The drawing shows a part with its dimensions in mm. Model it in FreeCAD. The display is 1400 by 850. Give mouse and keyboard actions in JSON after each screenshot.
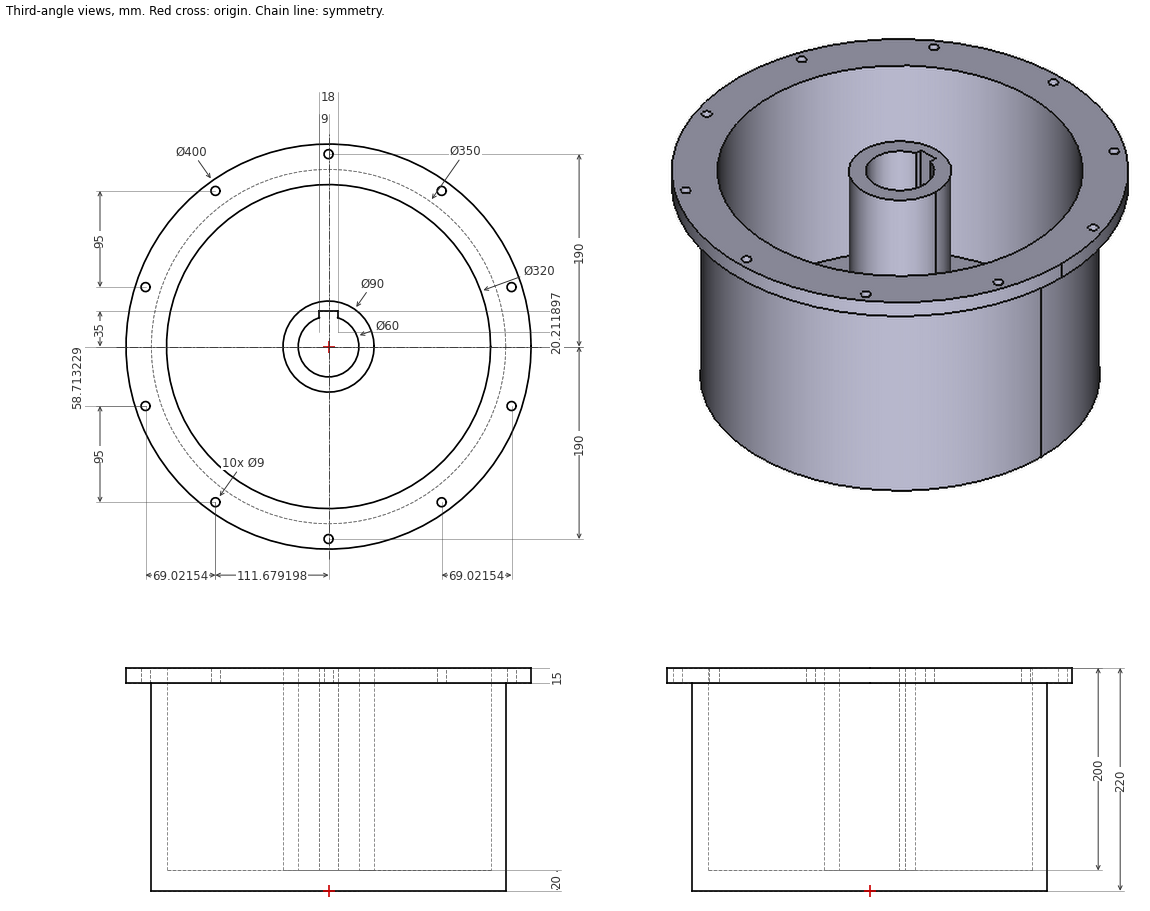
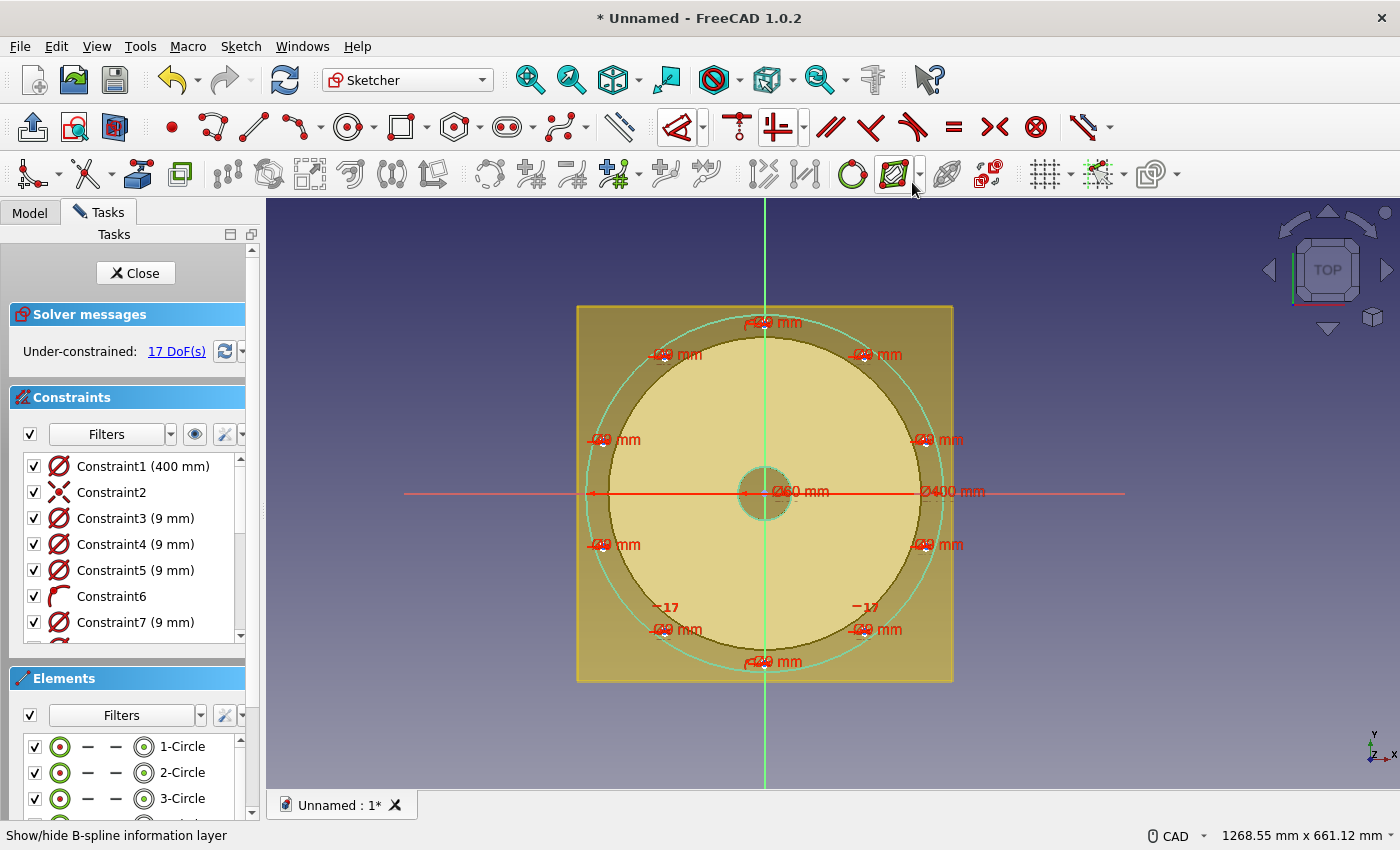
{"action": "left_click", "coordinate": [603, 547]}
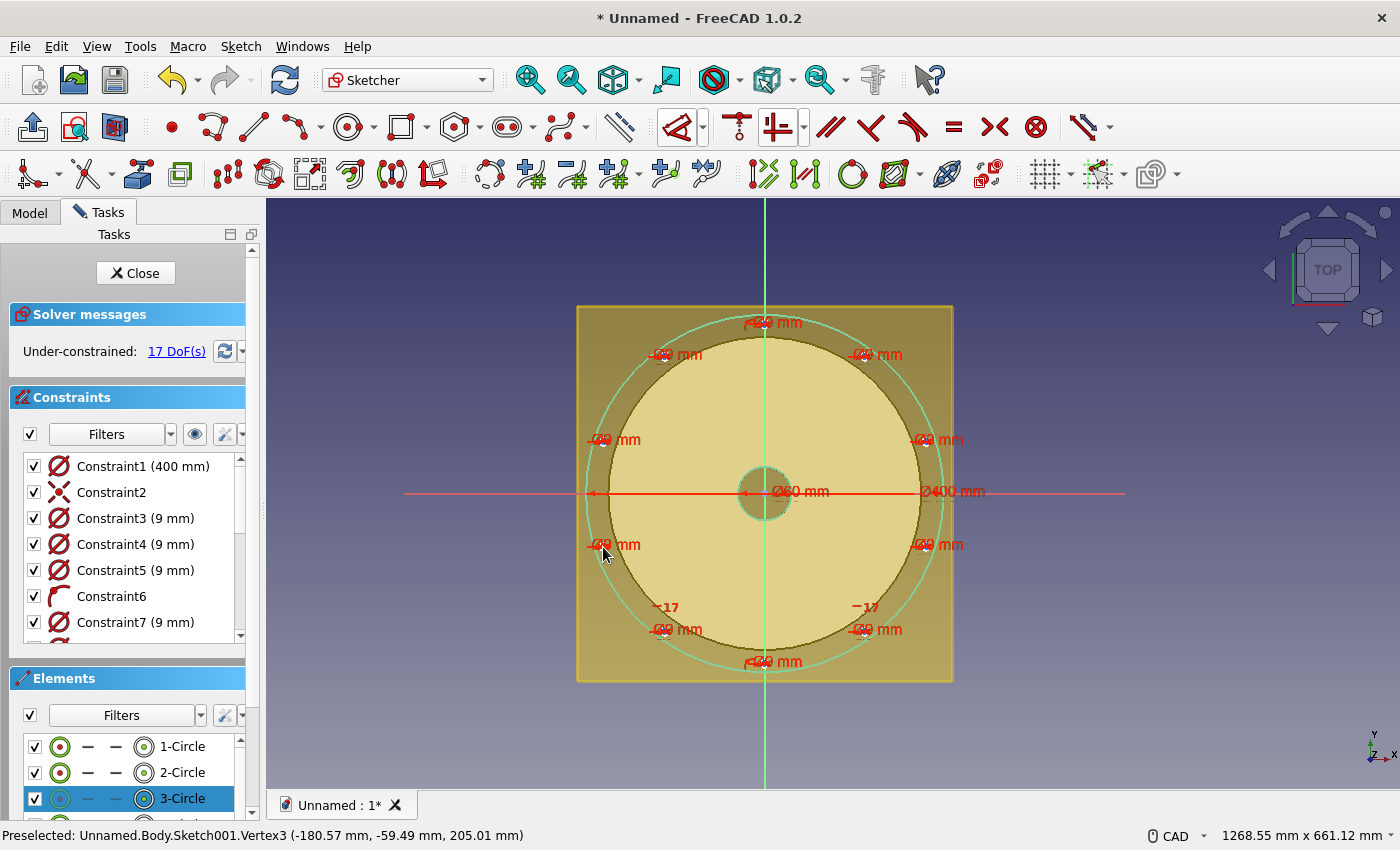
{"action": "left_click", "coordinate": [926, 547]}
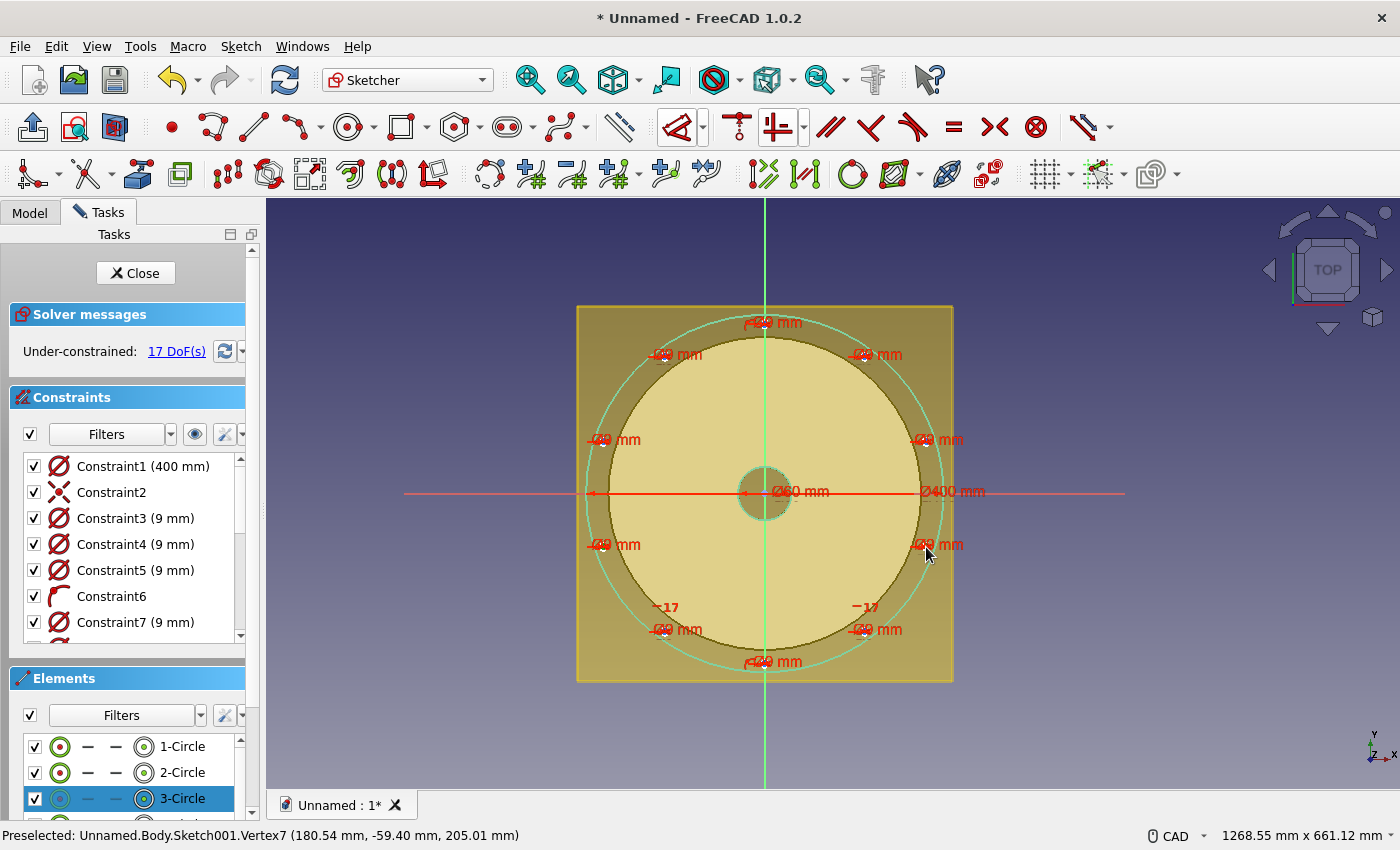
{"action": "left_click", "coordinate": [804, 128]}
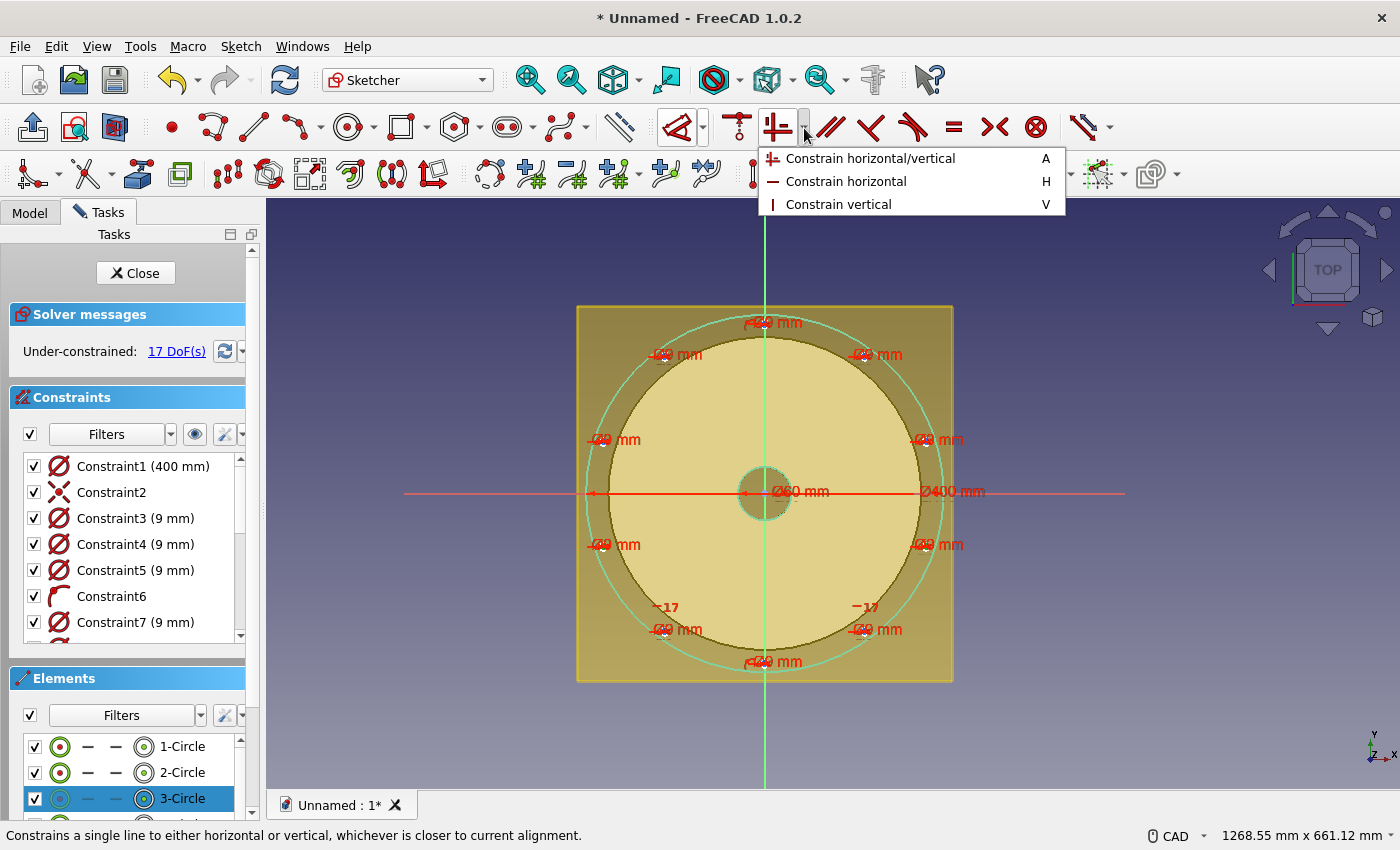
{"action": "left_click", "coordinate": [912, 182]}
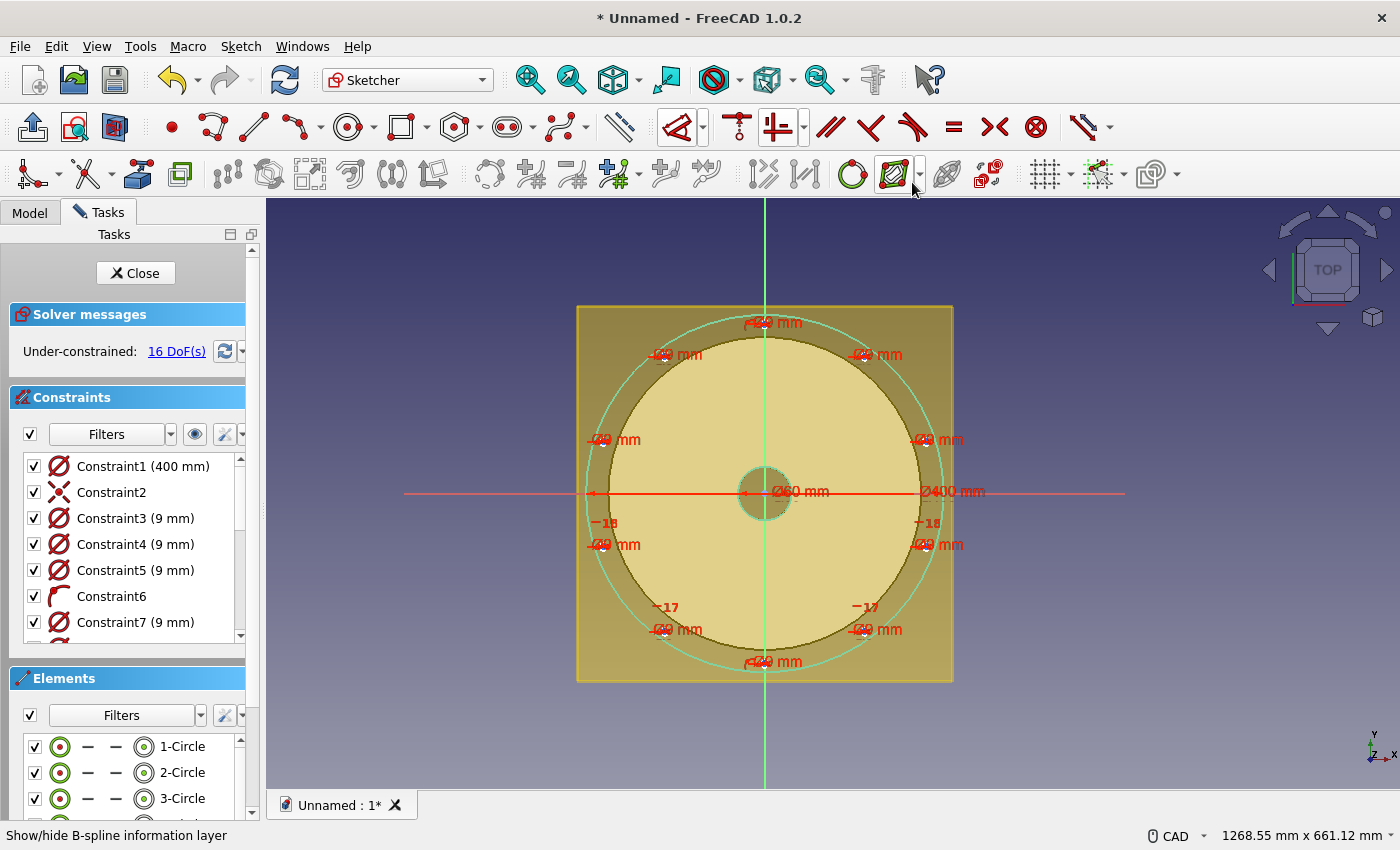
{"action": "left_click", "coordinate": [603, 547]}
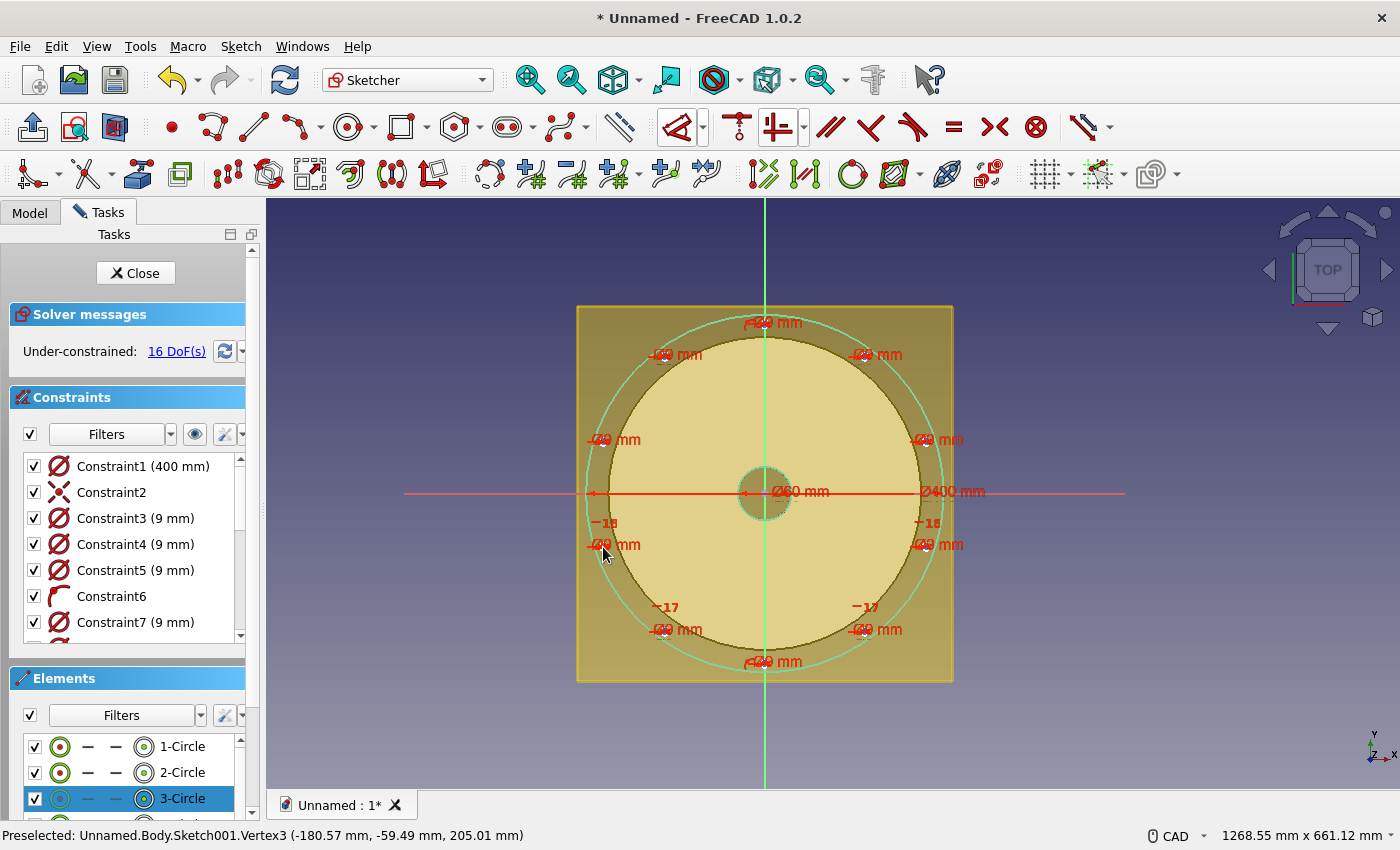
{"action": "left_click", "coordinate": [603, 442]}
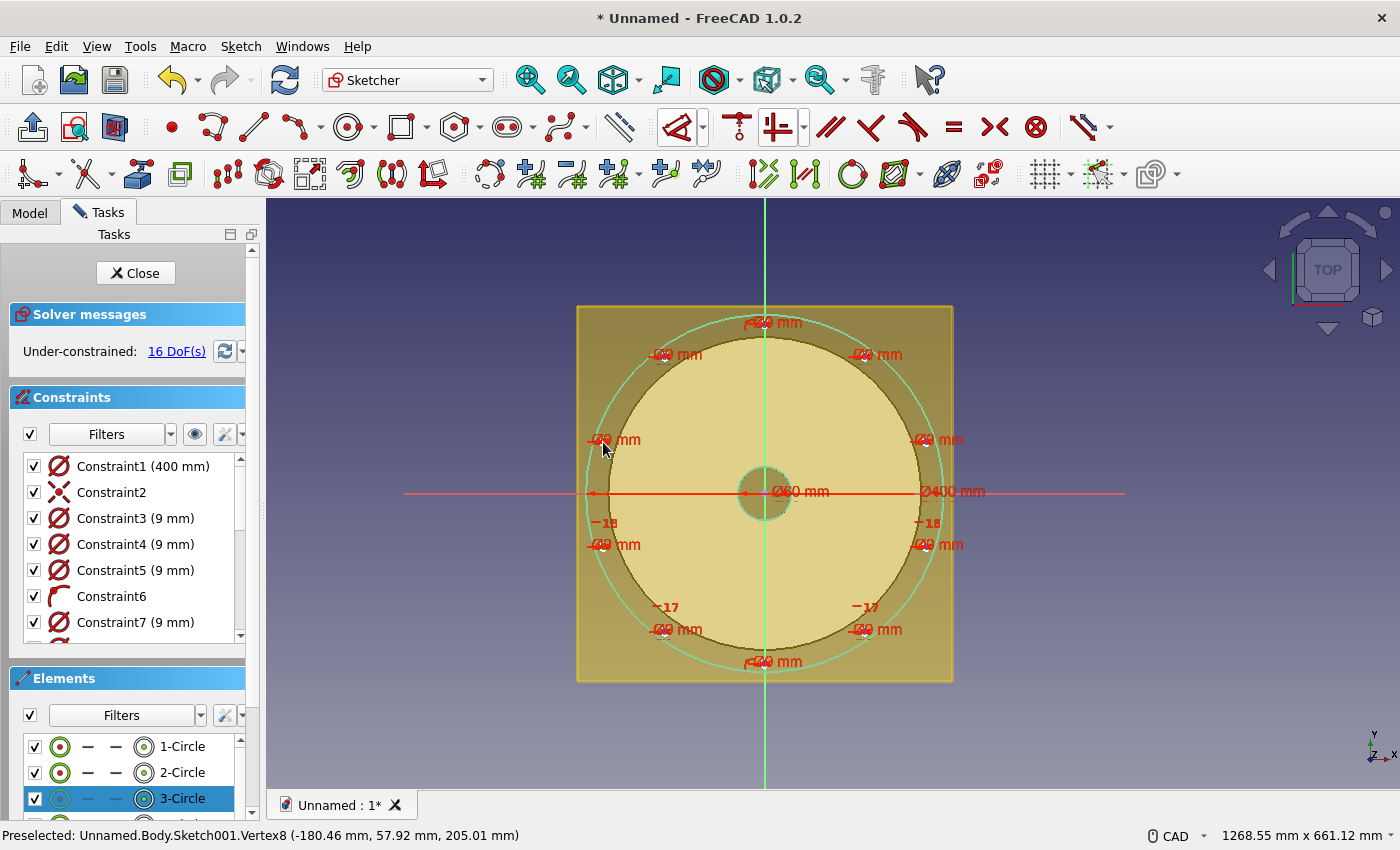
{"action": "key", "text": "v"}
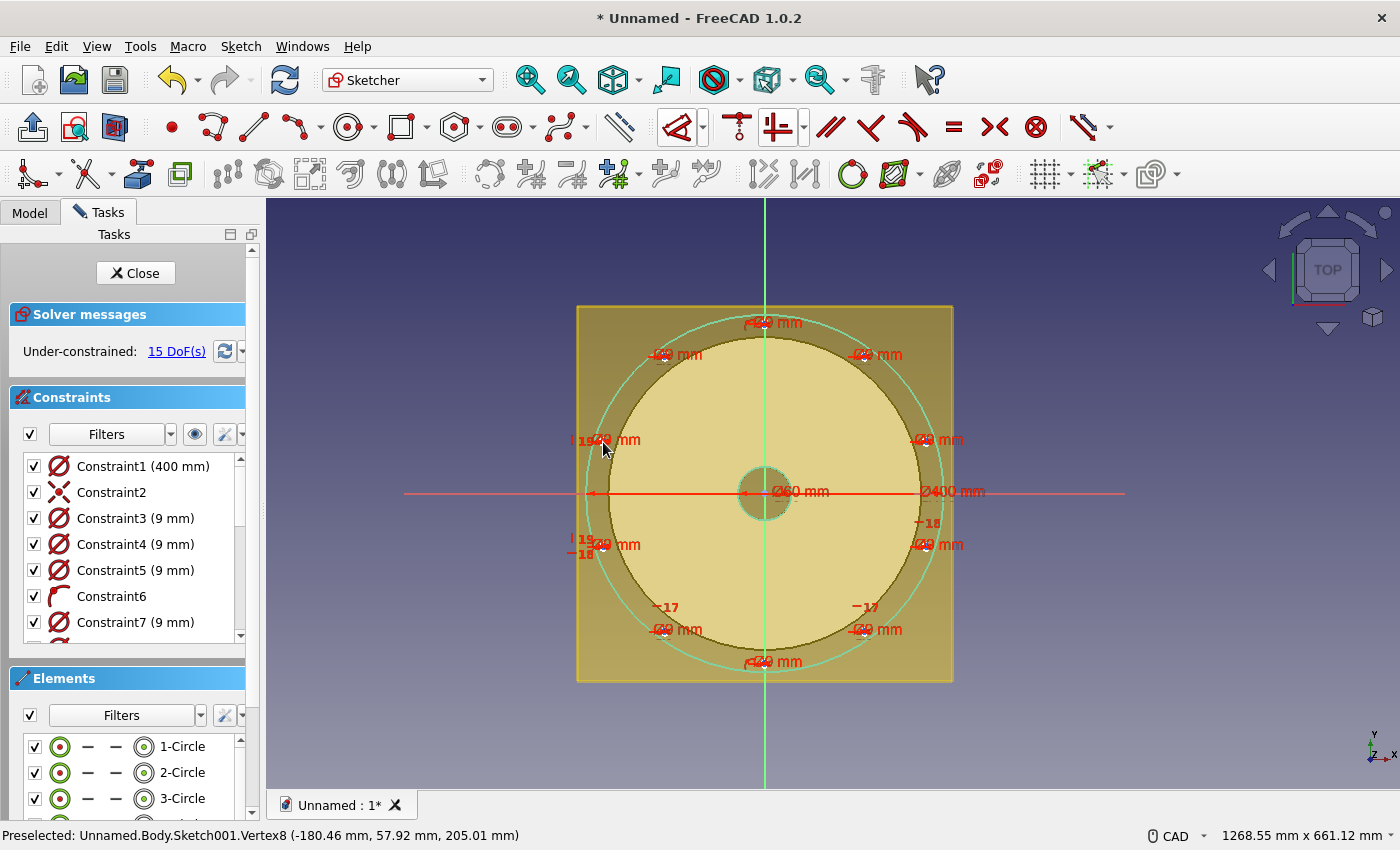
{"action": "left_click", "coordinate": [665, 632]}